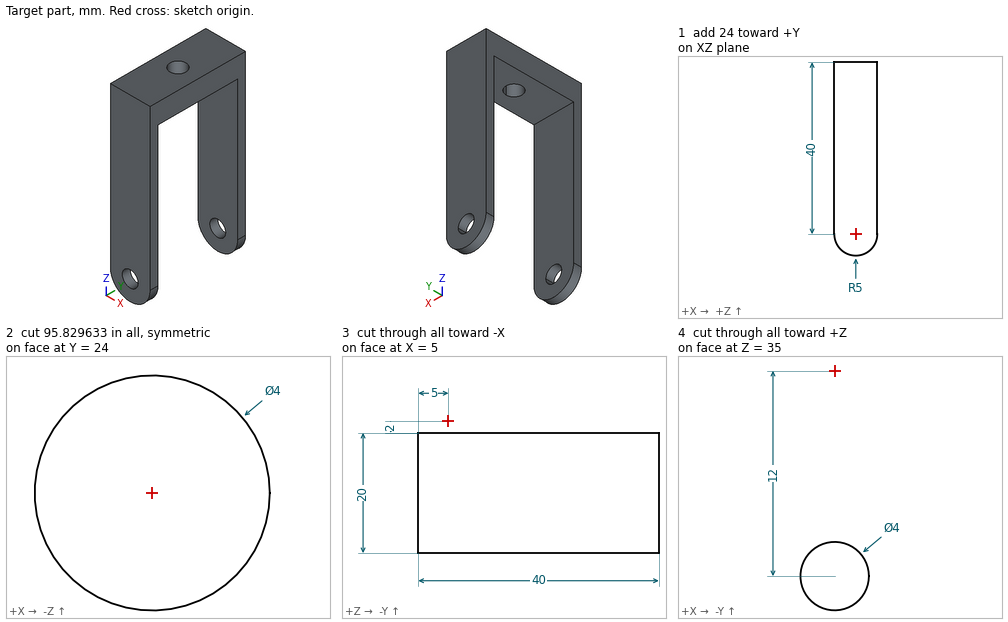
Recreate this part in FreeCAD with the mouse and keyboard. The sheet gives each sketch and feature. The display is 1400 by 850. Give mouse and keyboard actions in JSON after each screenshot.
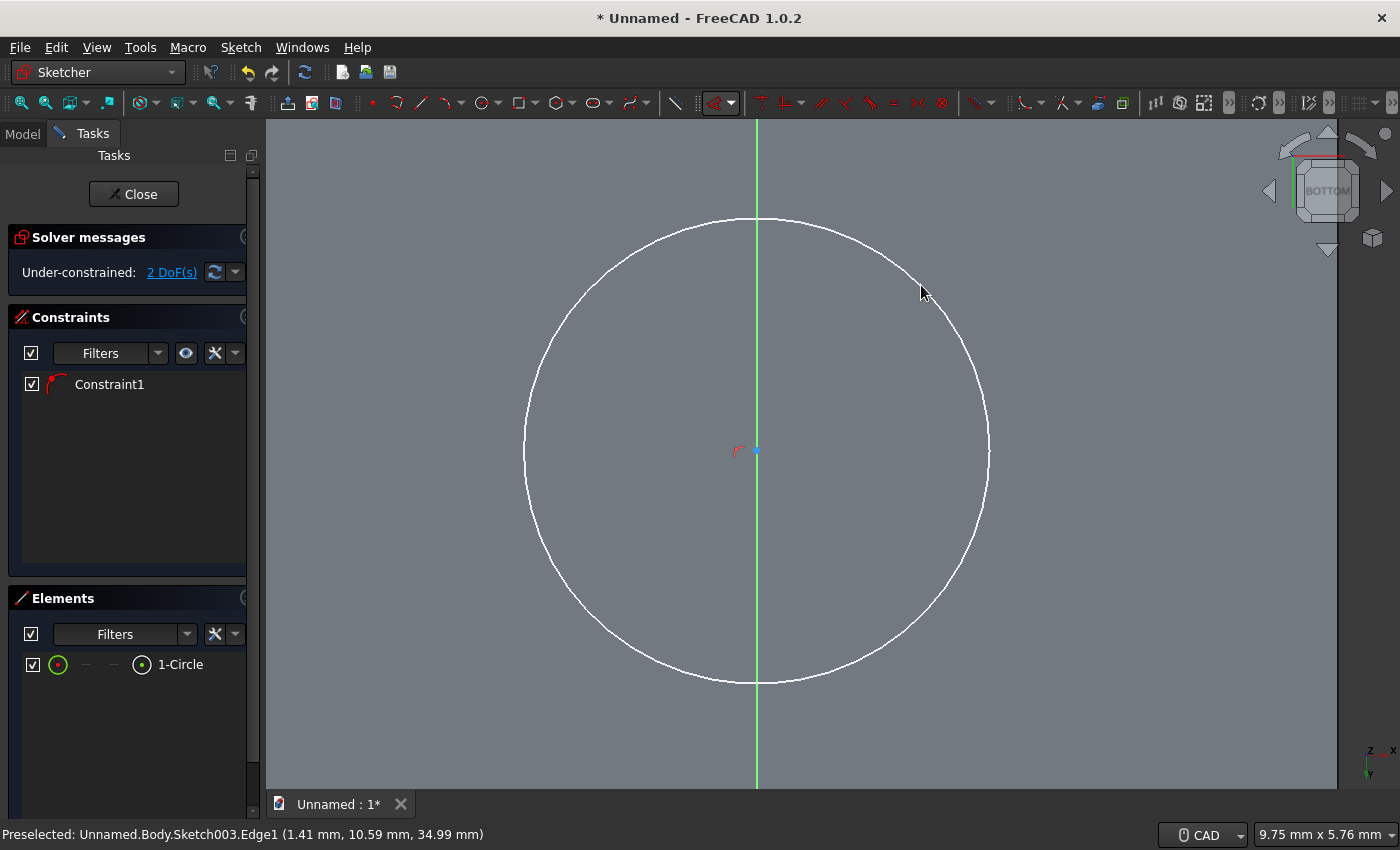
{"action": "left_click", "coordinate": [921, 286]}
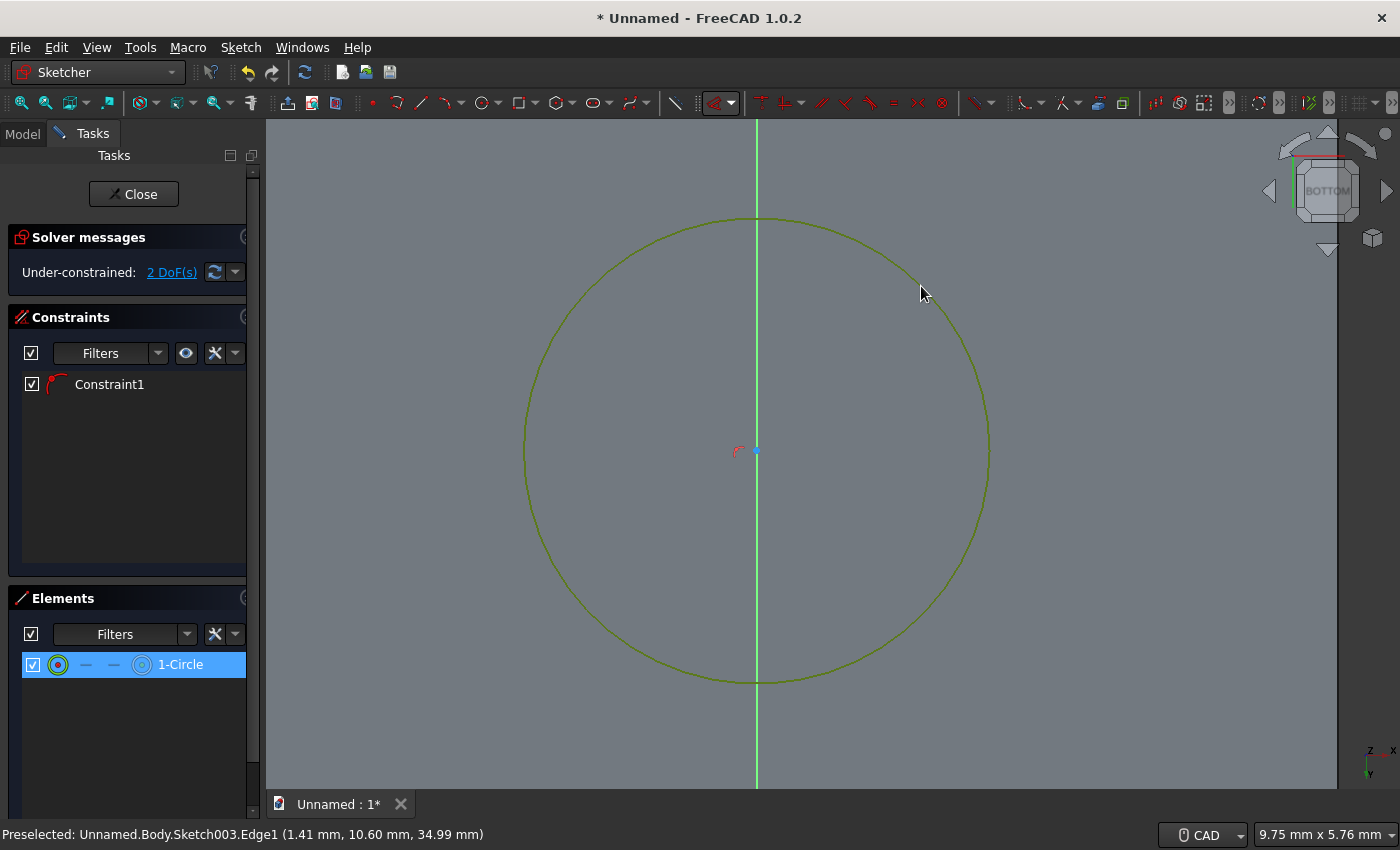
{"action": "key", "text": "k o"}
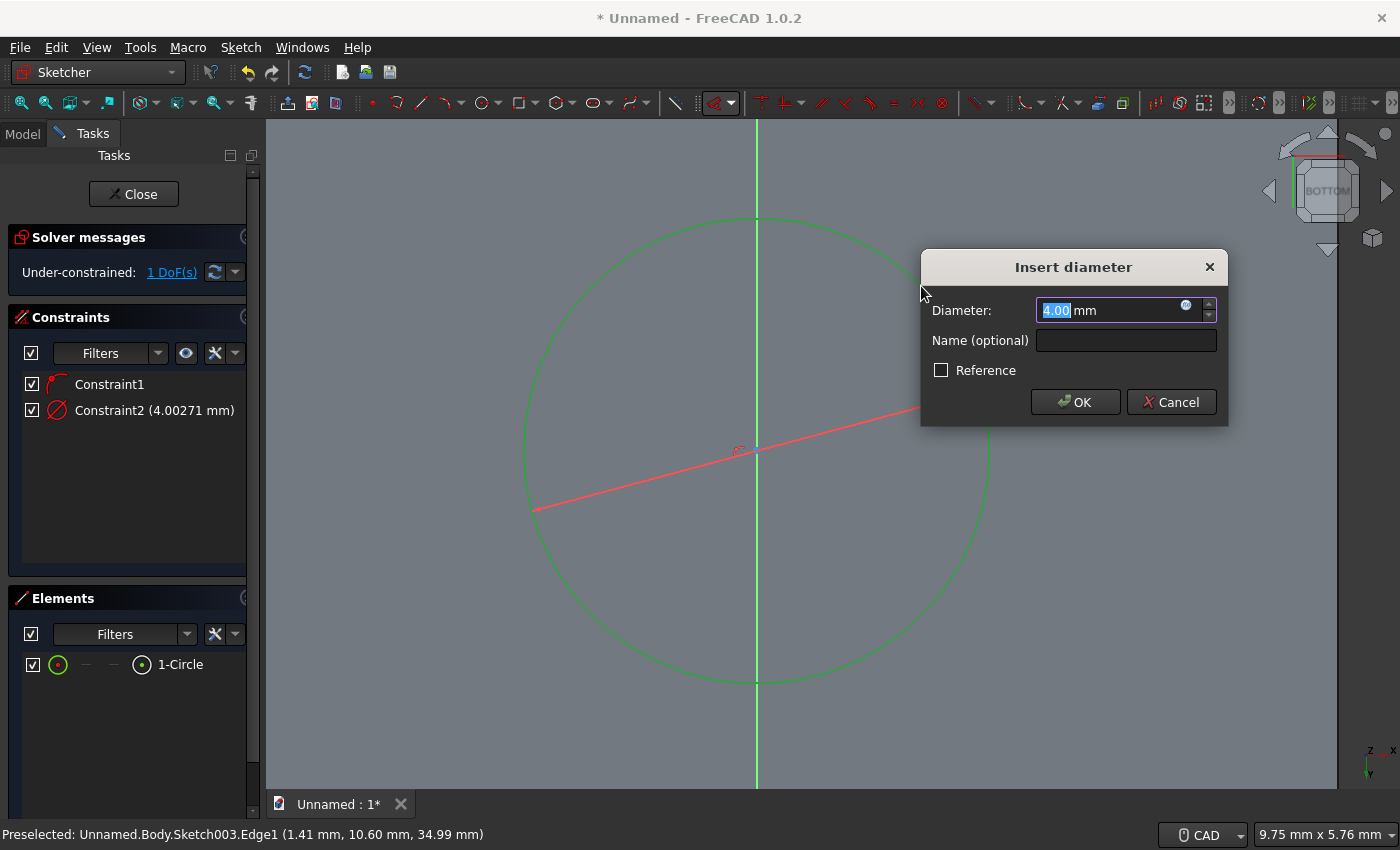
{"action": "type", "text": "4"}
{"action": "key", "text": "Return"}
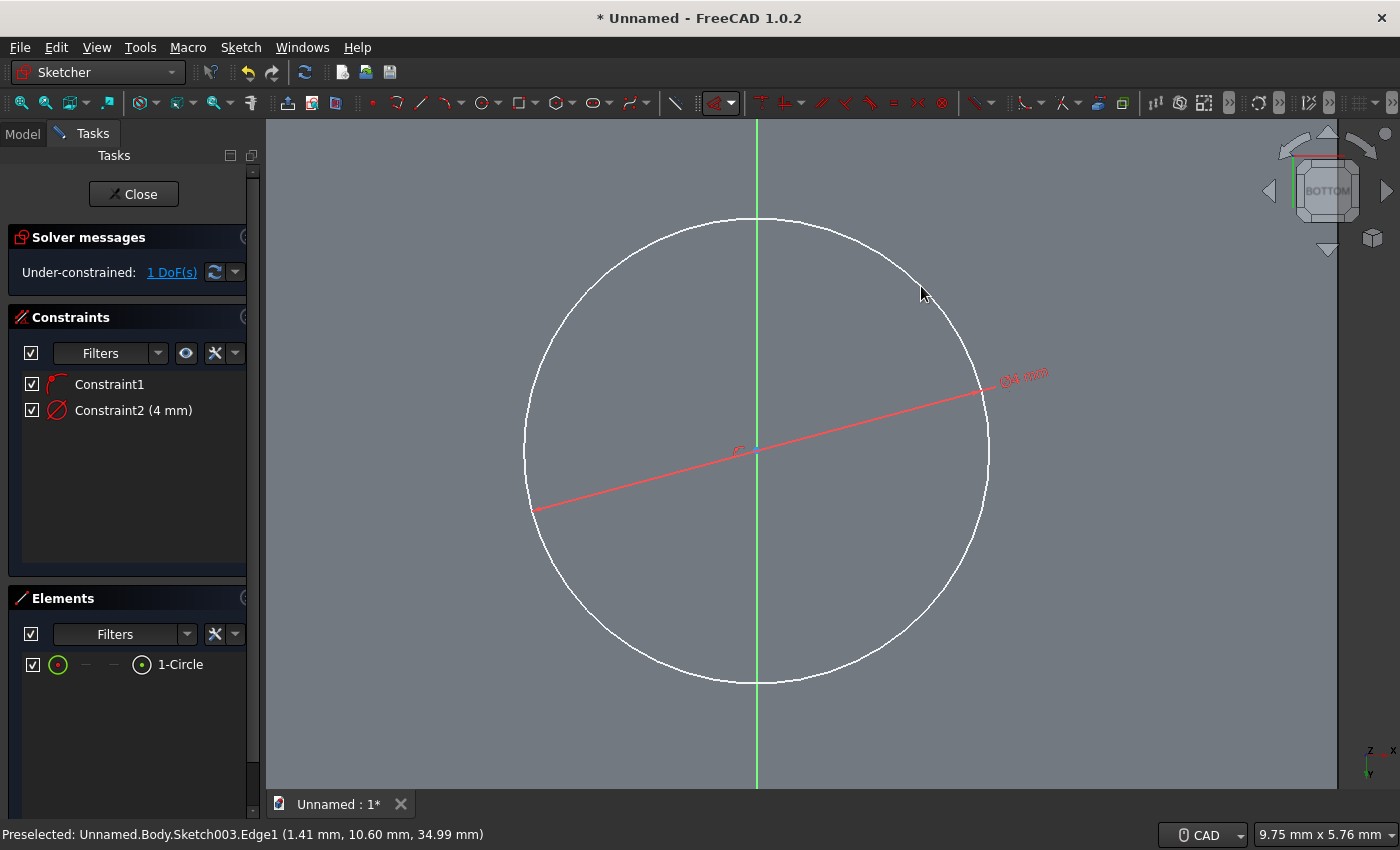
{"action": "left_click", "coordinate": [757, 451]}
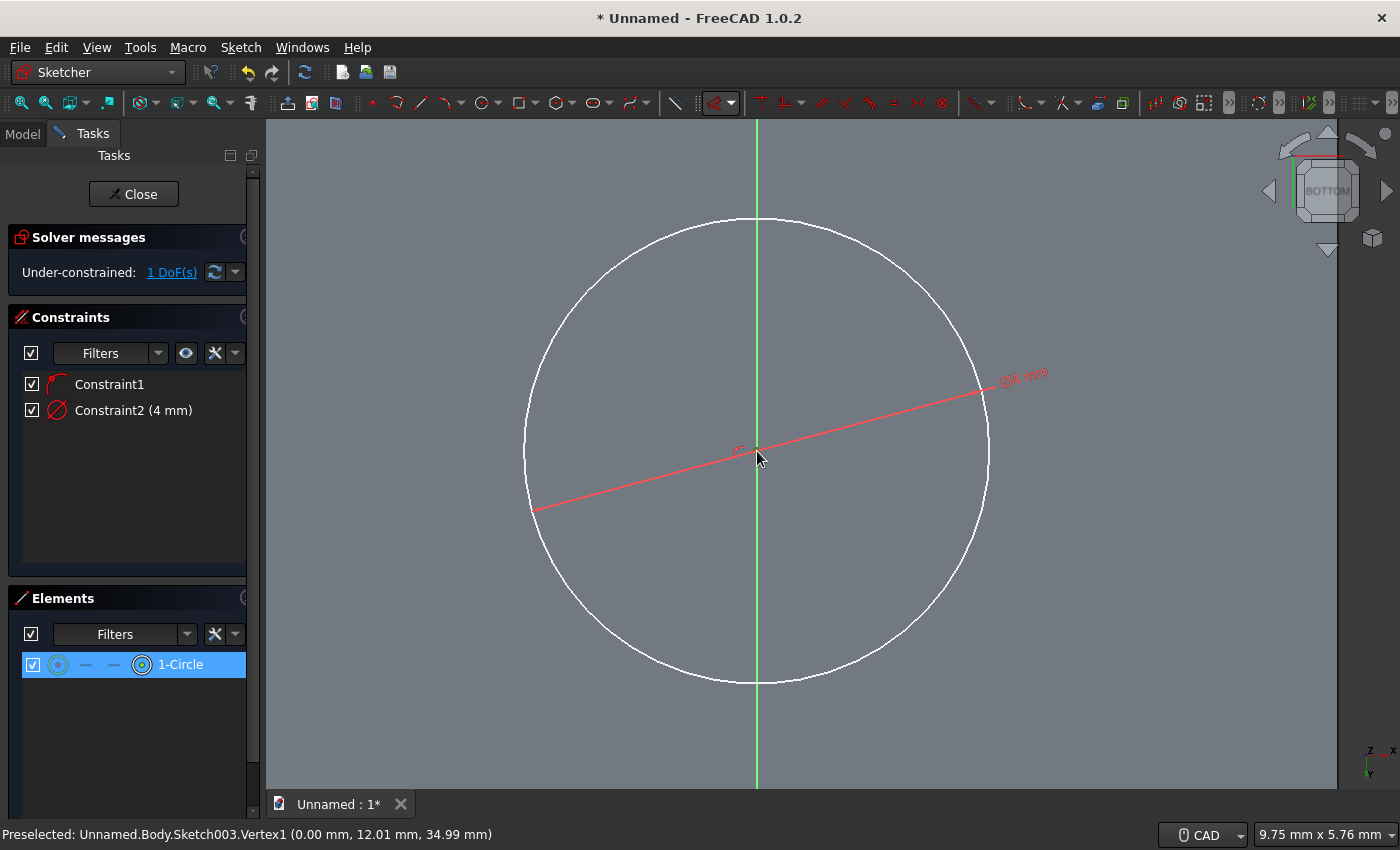
{"action": "key", "text": "i"}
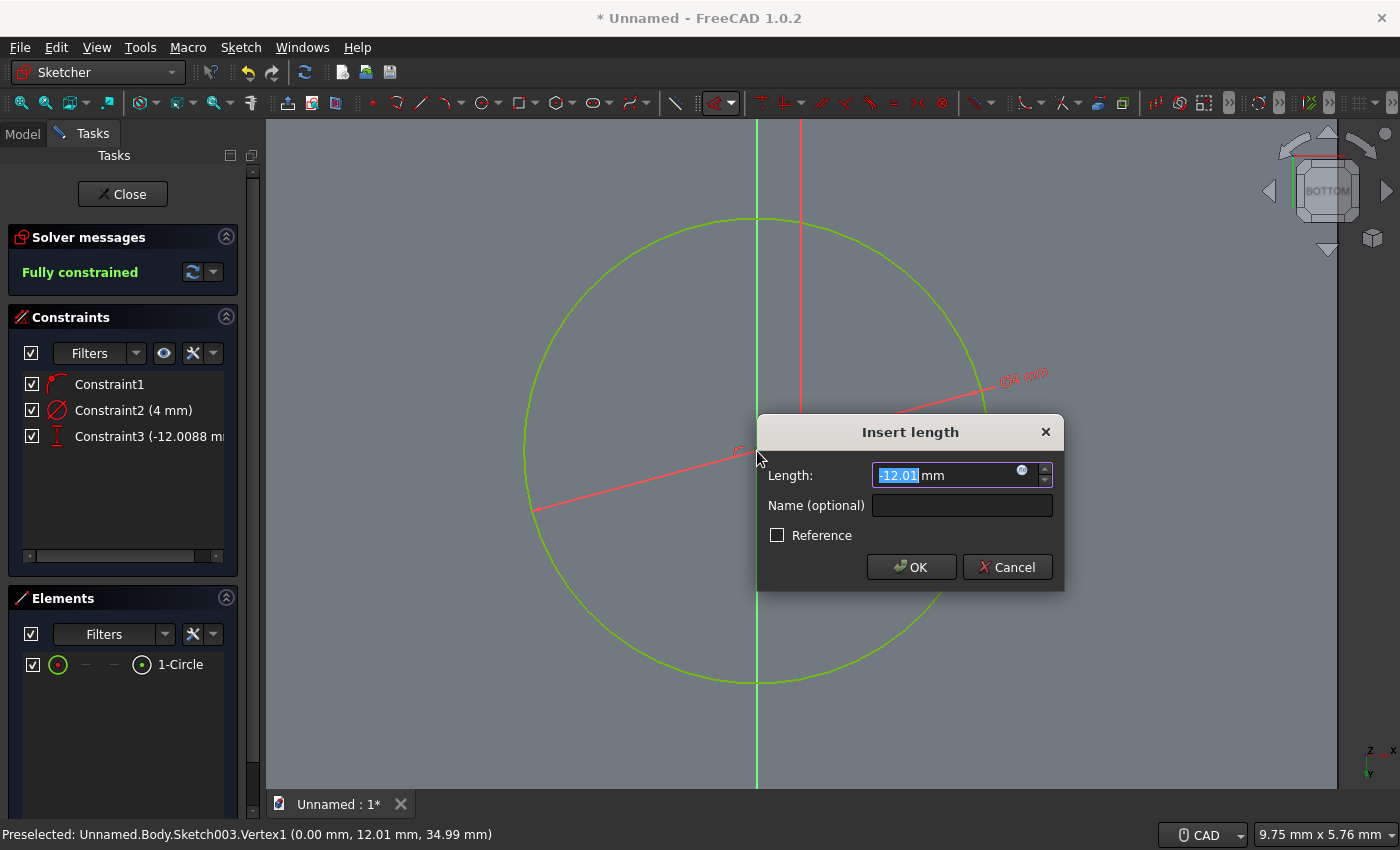
{"action": "type", "text": "-12"}
{"action": "key", "text": "Return"}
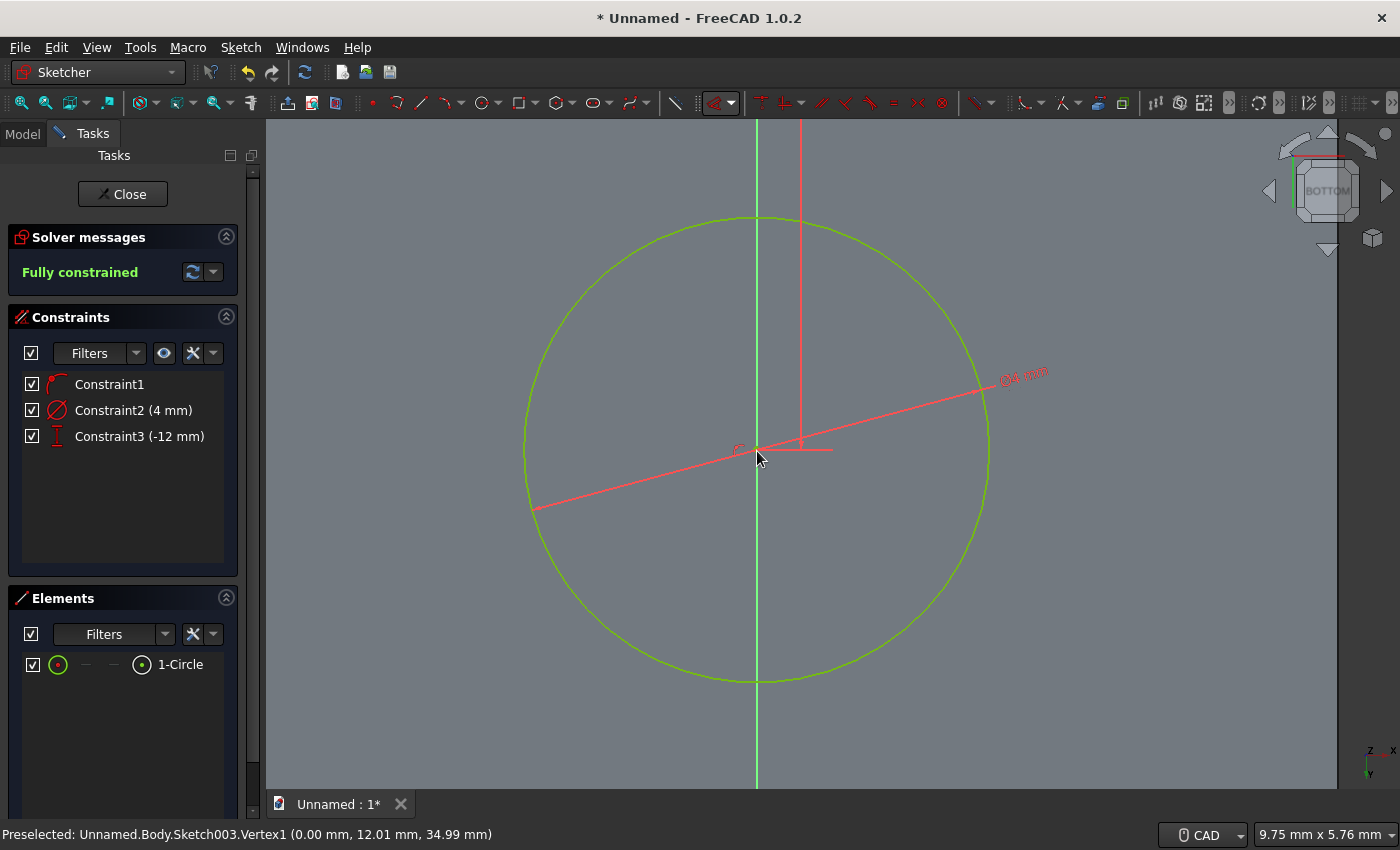
{"action": "left_click", "coordinate": [123, 194]}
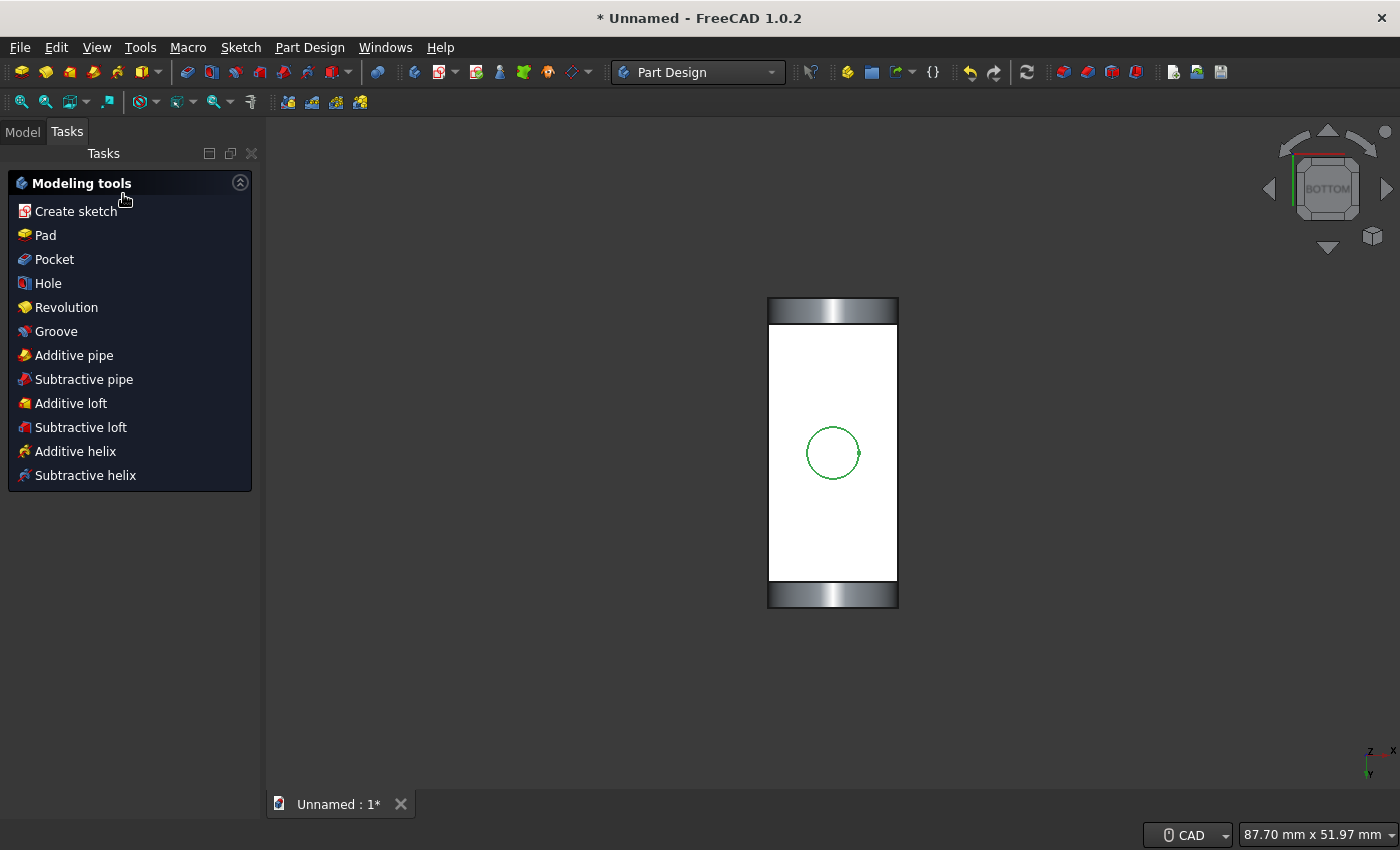
{"action": "left_click", "coordinate": [188, 72]}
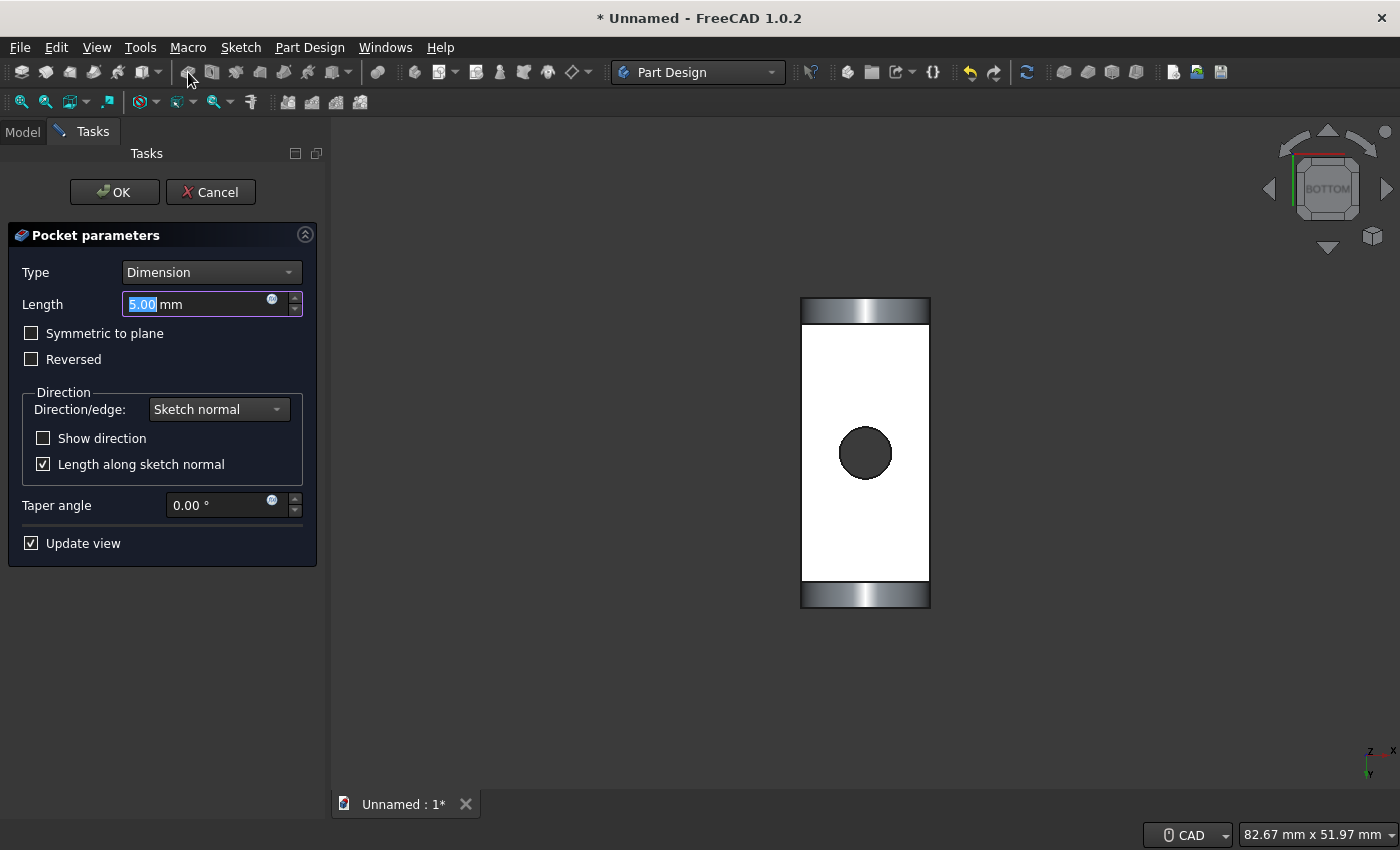
{"action": "left_click", "coordinate": [212, 272]}